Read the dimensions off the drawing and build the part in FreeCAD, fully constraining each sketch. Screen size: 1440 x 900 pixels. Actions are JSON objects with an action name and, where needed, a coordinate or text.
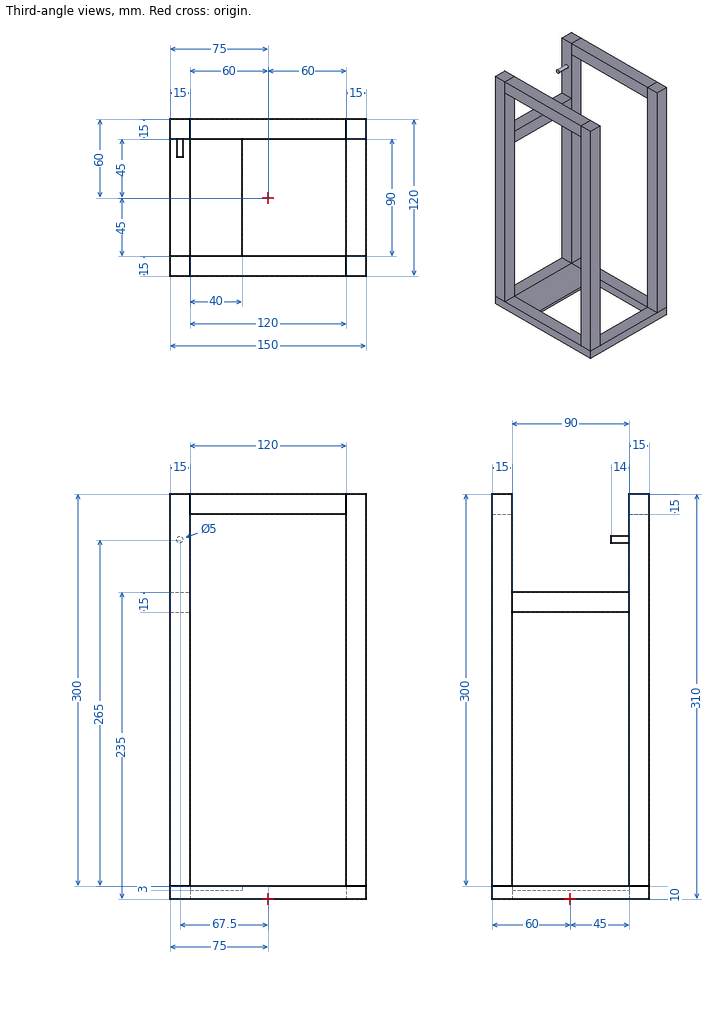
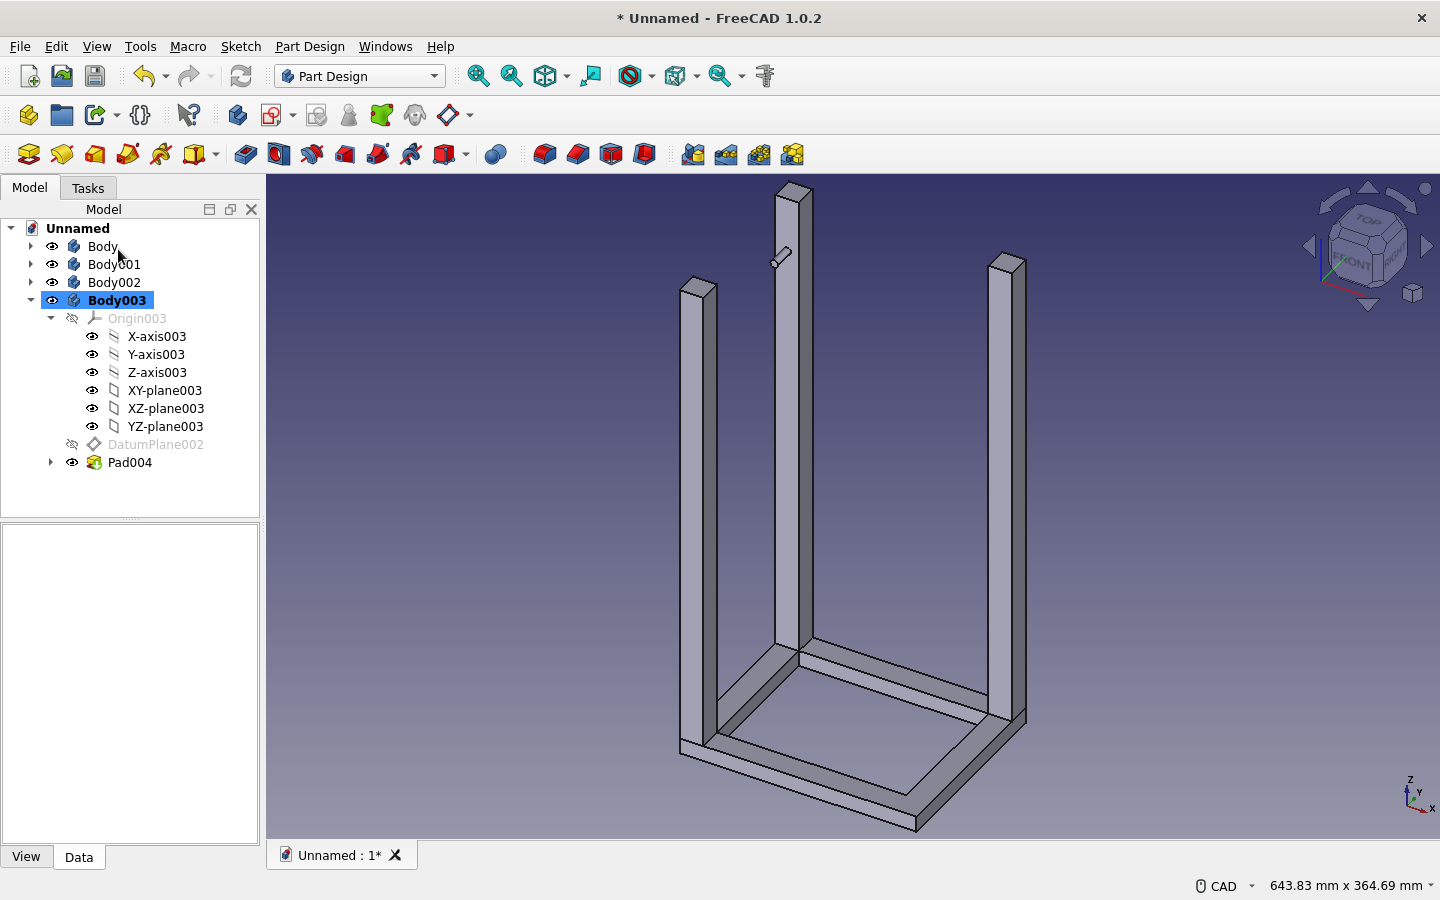
{"action": "left_click", "coordinate": [238, 116]}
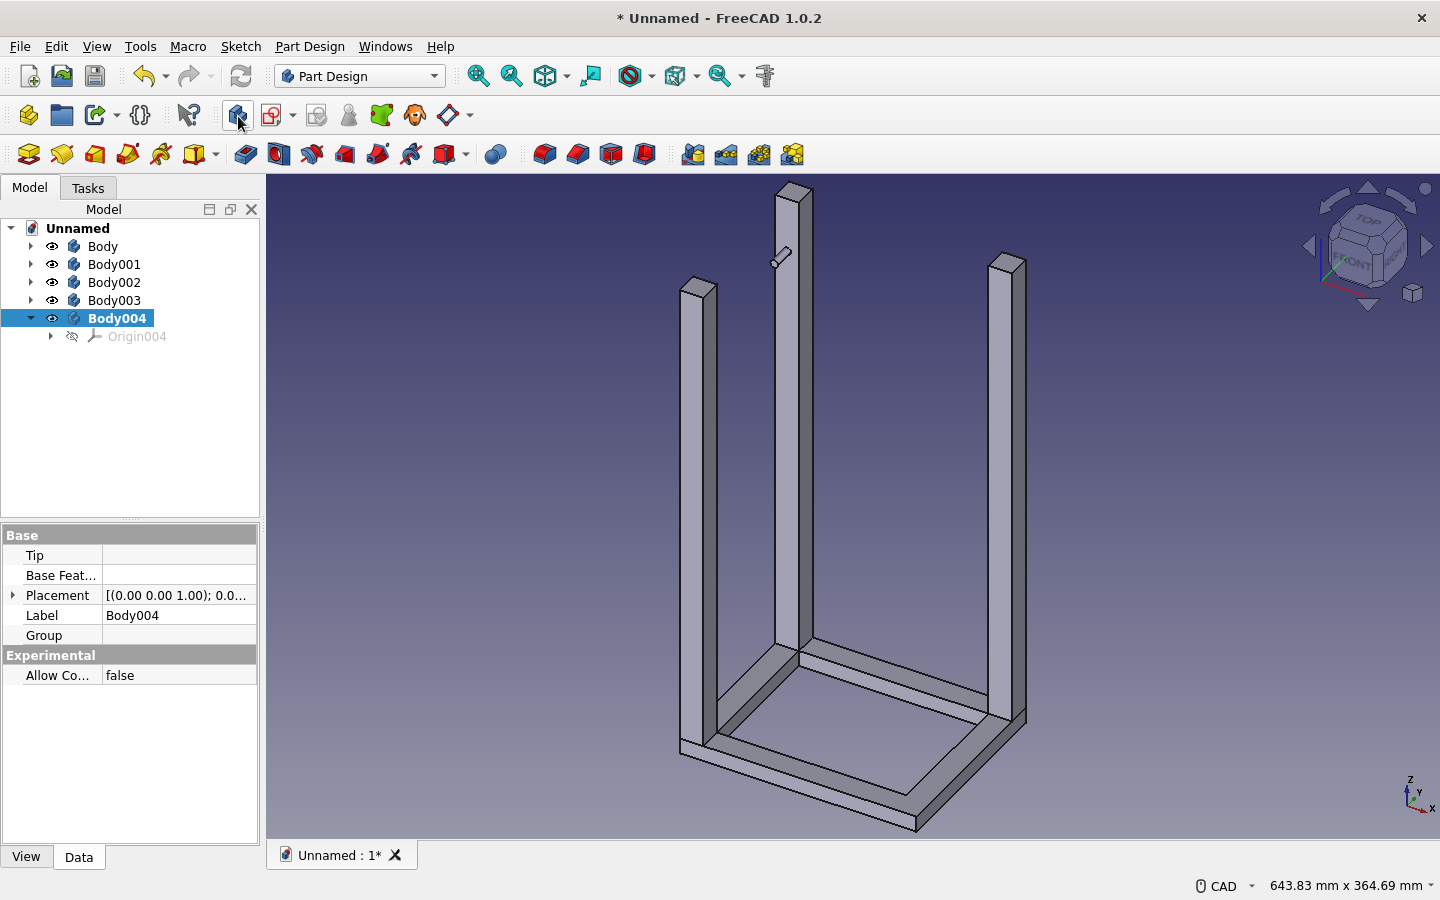
{"action": "left_click", "coordinate": [51, 336]}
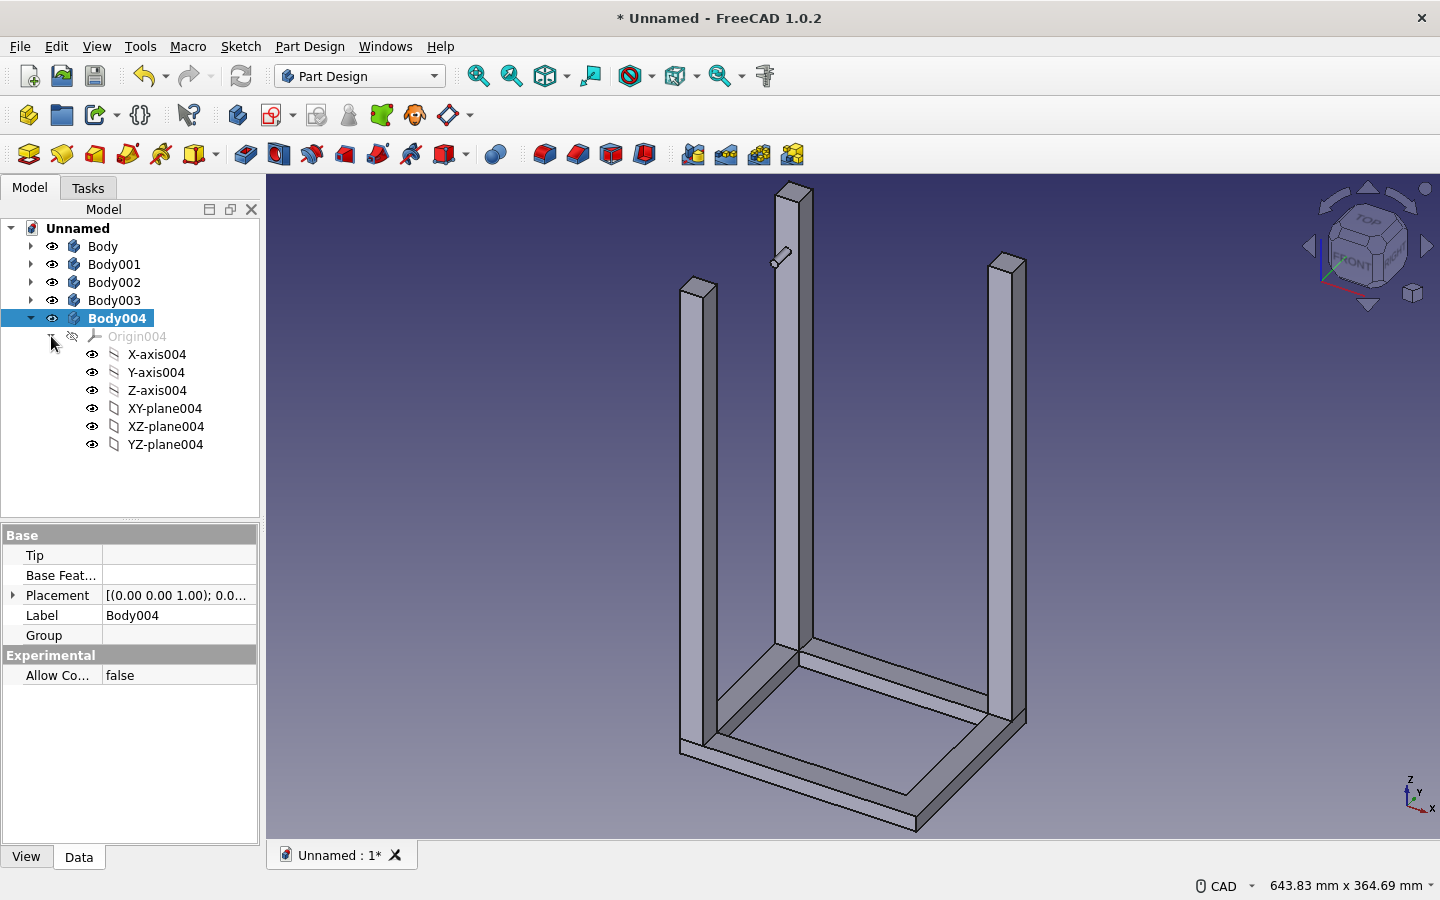
{"action": "left_click", "coordinate": [137, 408]}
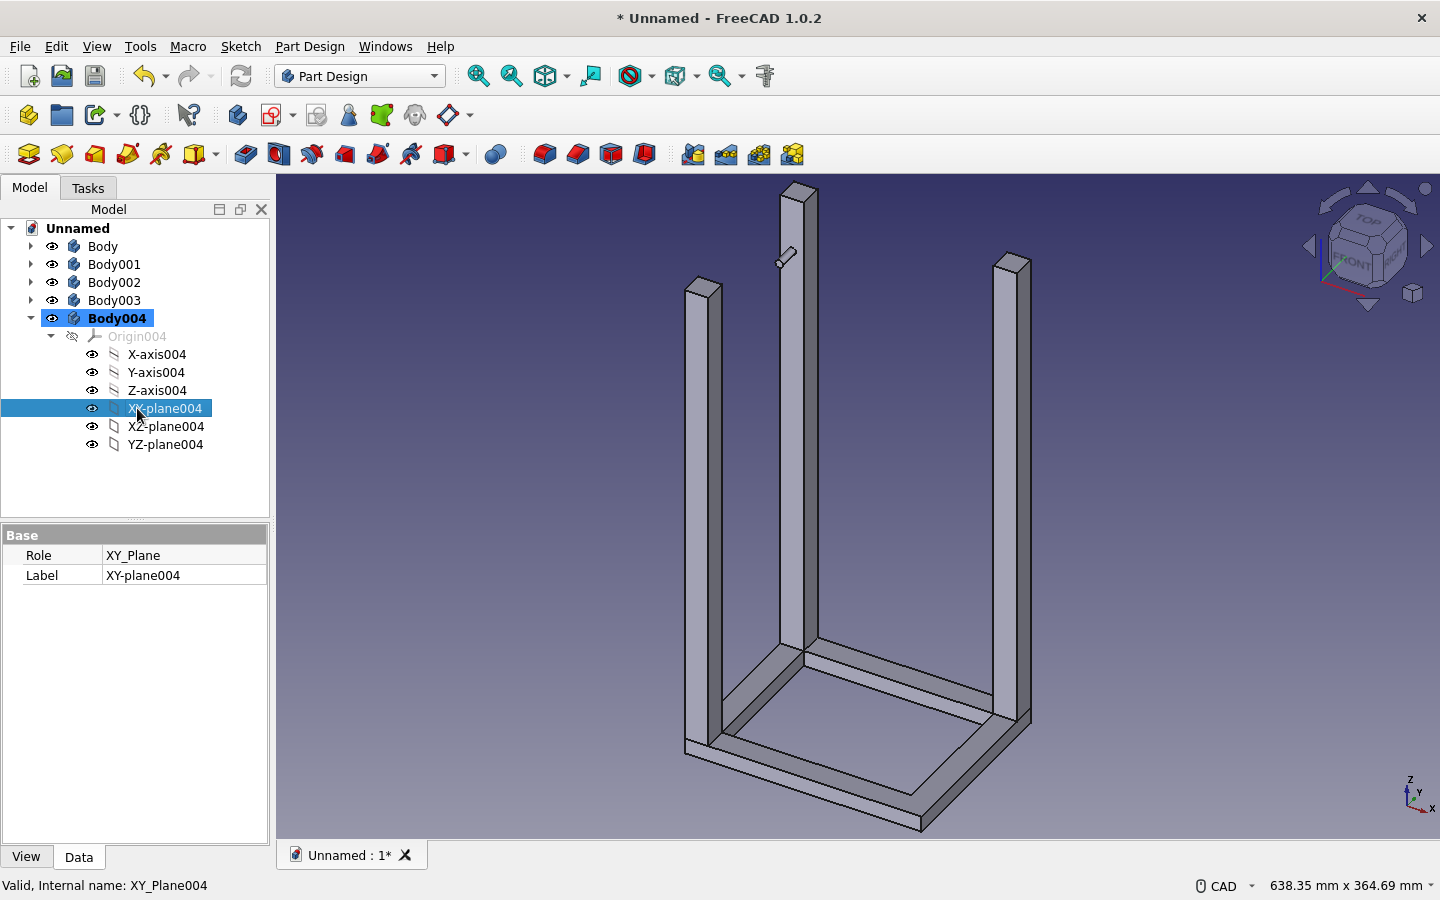
{"action": "left_click", "coordinate": [448, 116]}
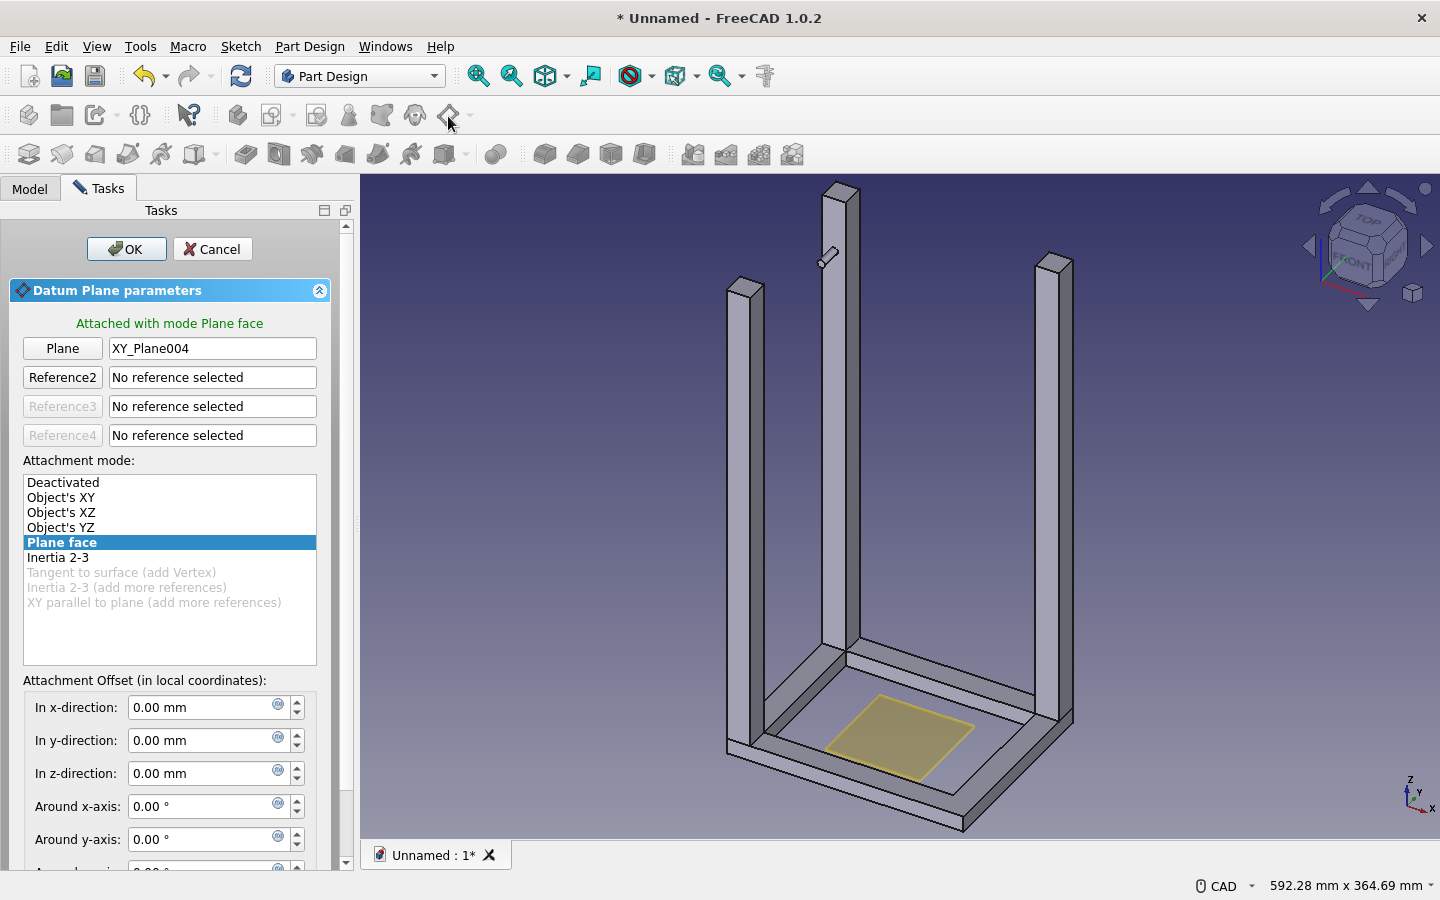
{"action": "triple_click", "coordinate": [210, 774]}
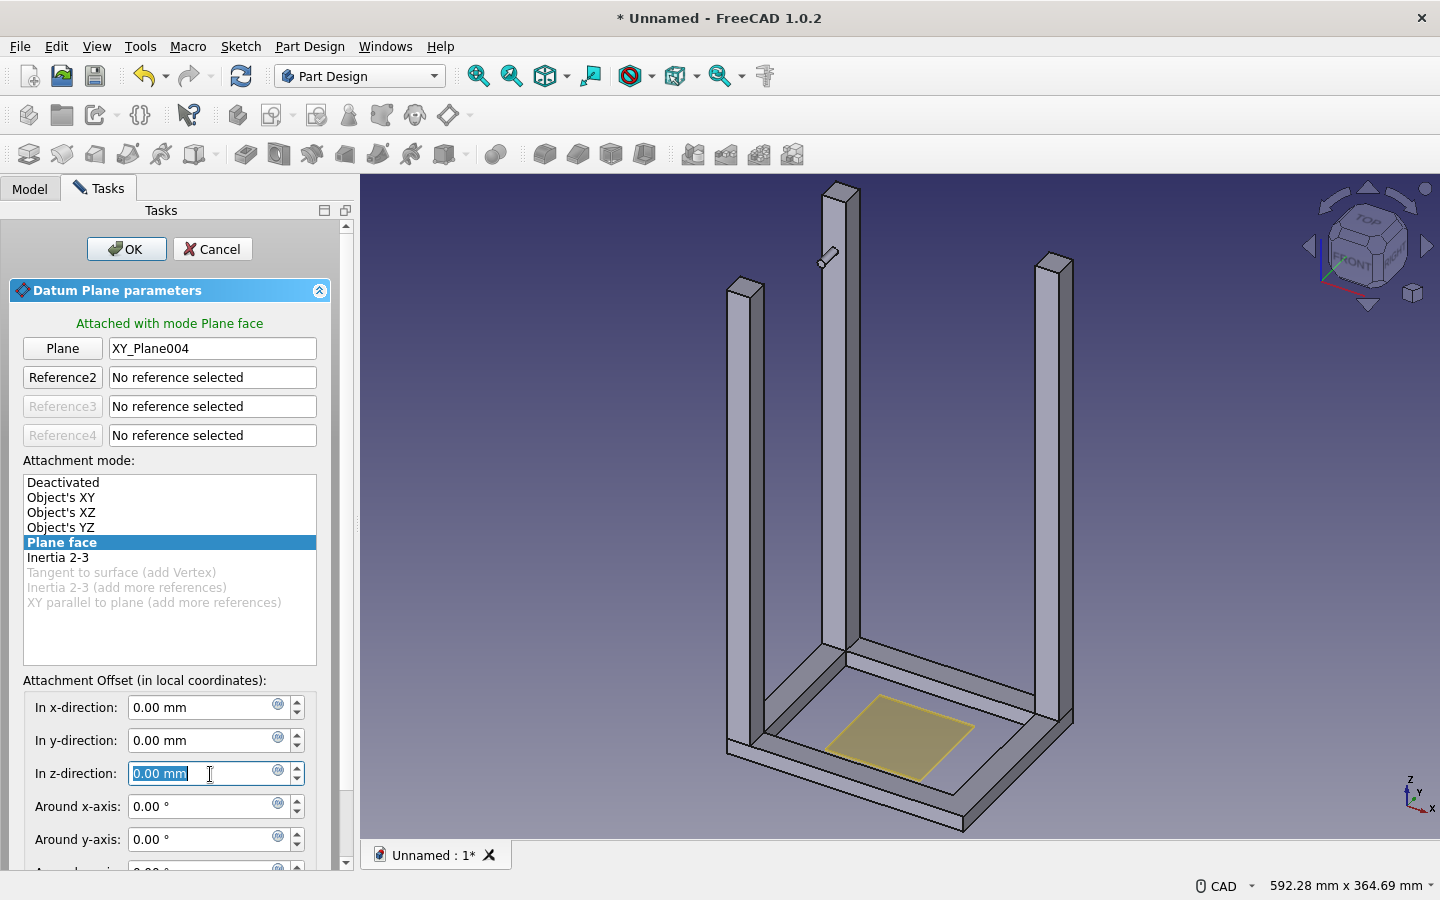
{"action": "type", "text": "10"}
{"action": "key", "text": "Tab"}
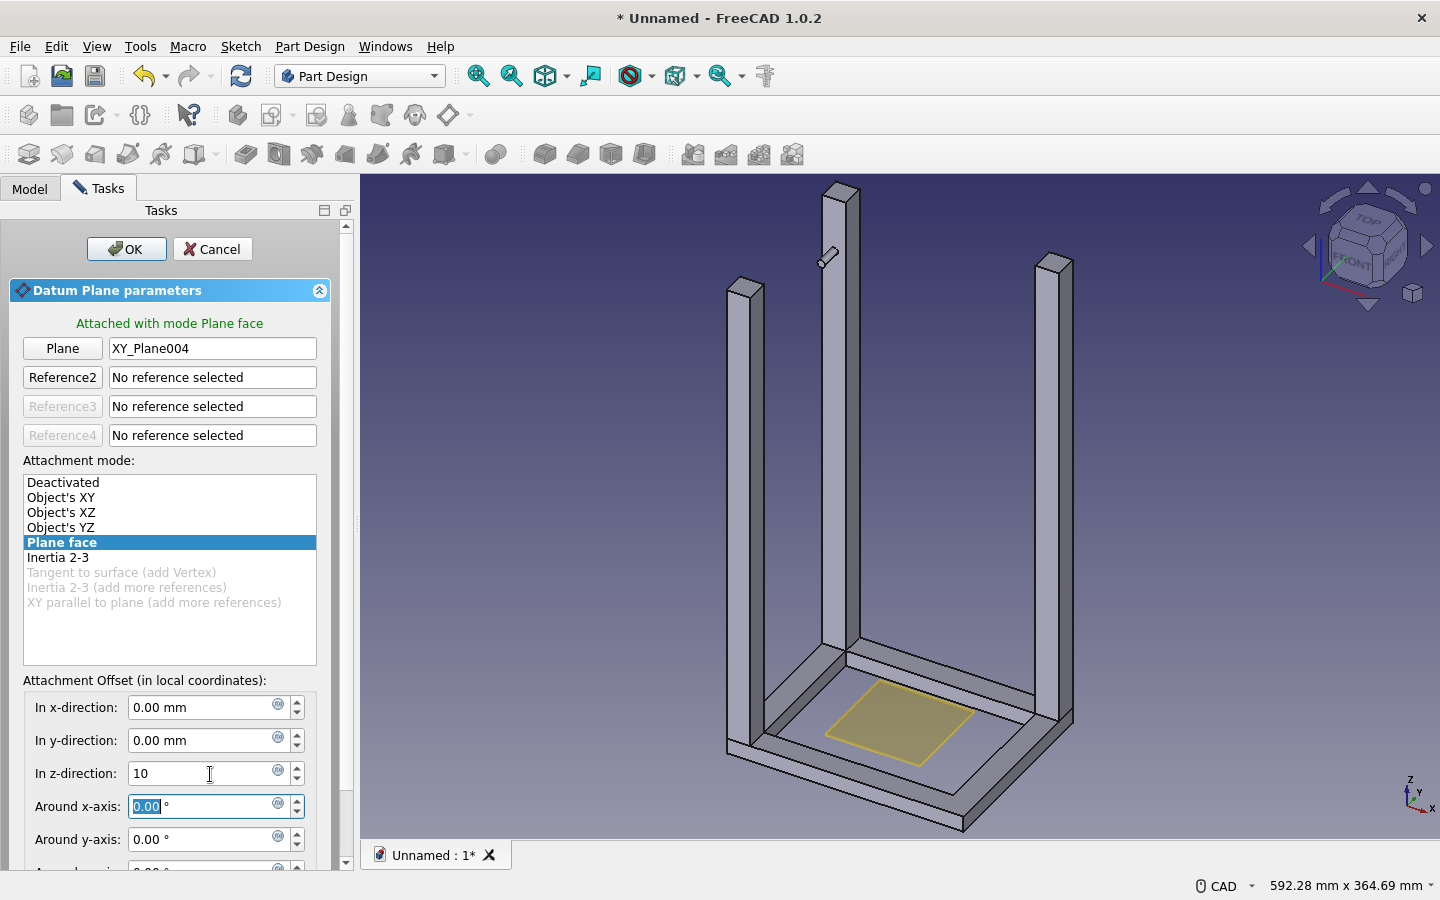
{"action": "left_click", "coordinate": [127, 249]}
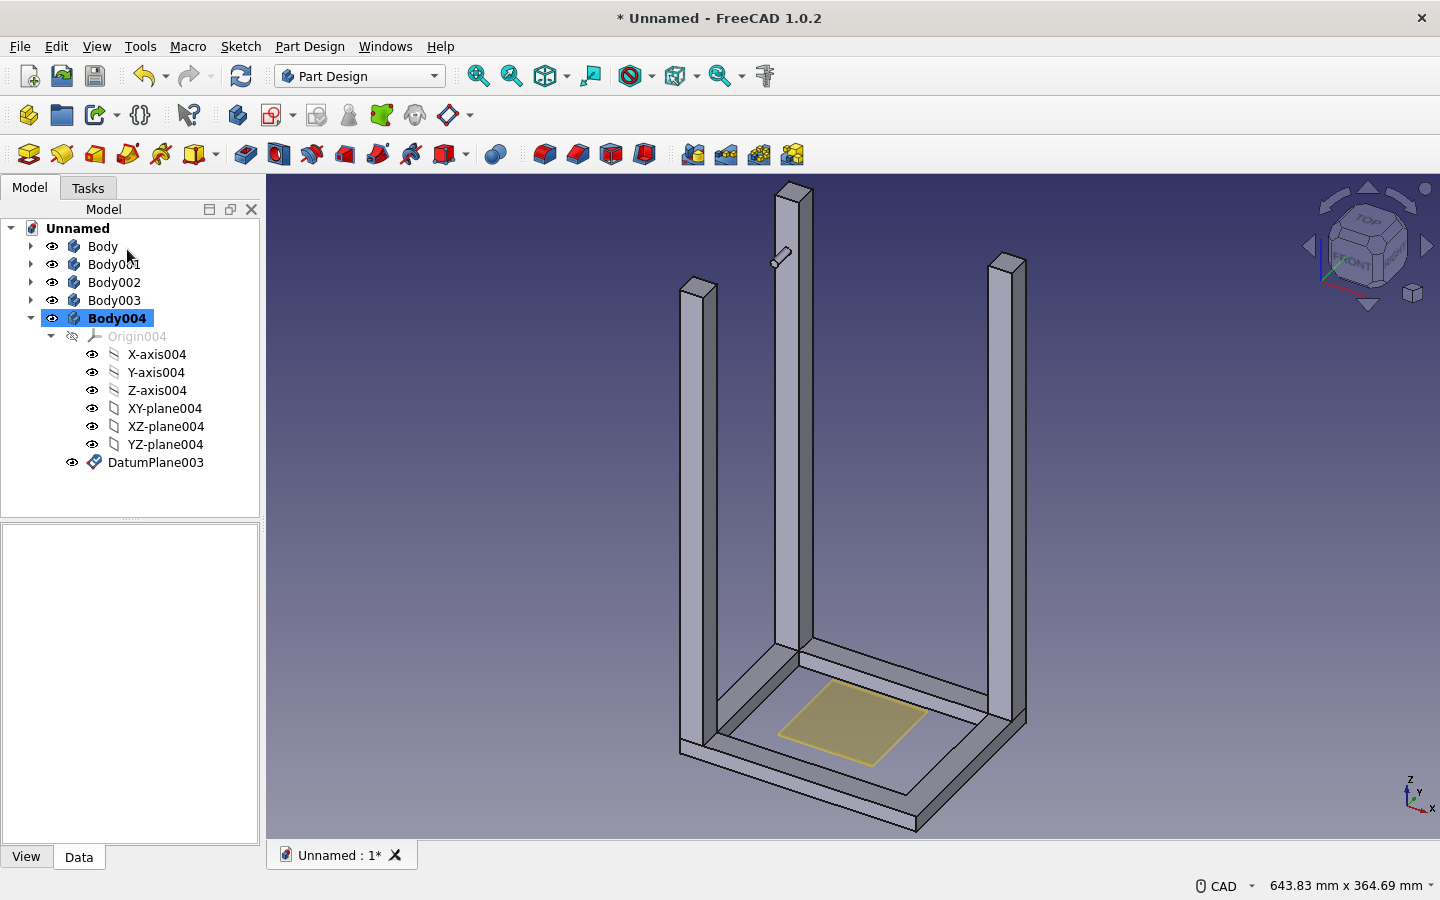
{"action": "left_click", "coordinate": [117, 462]}